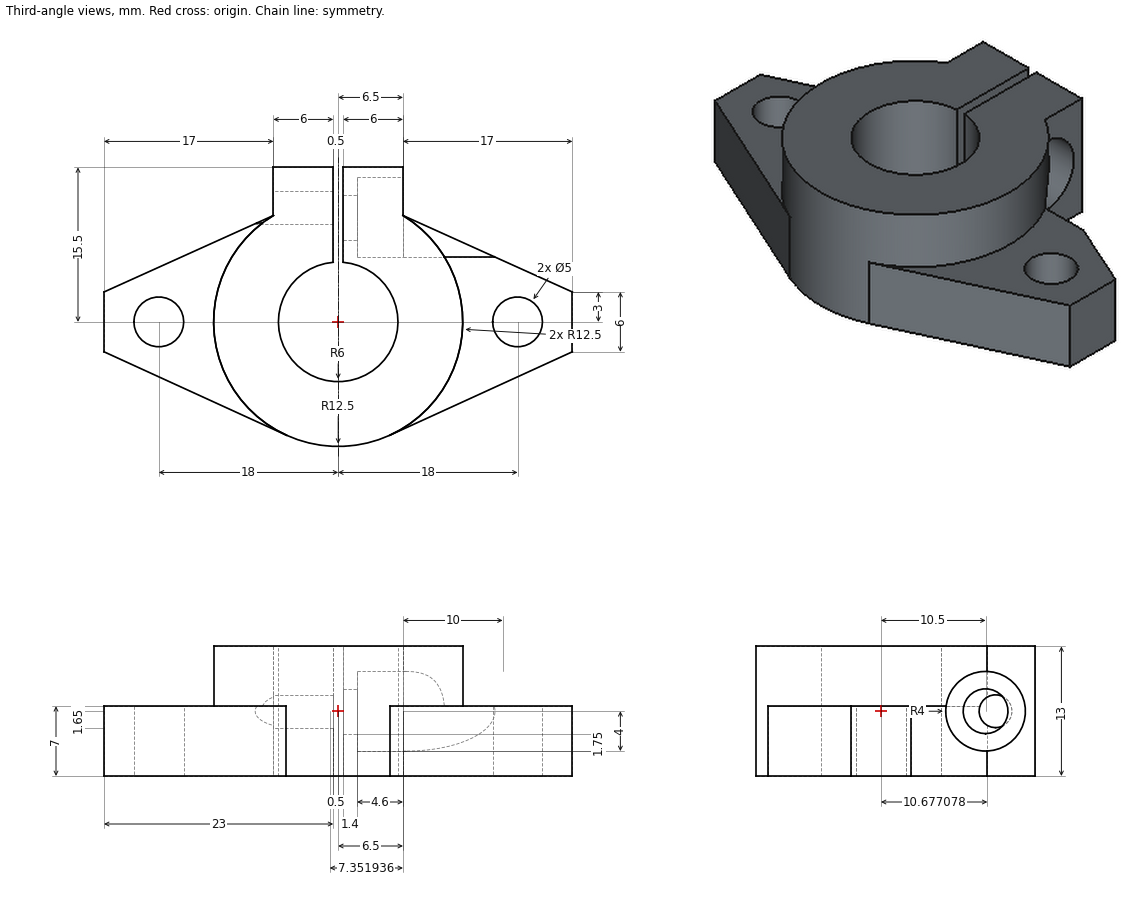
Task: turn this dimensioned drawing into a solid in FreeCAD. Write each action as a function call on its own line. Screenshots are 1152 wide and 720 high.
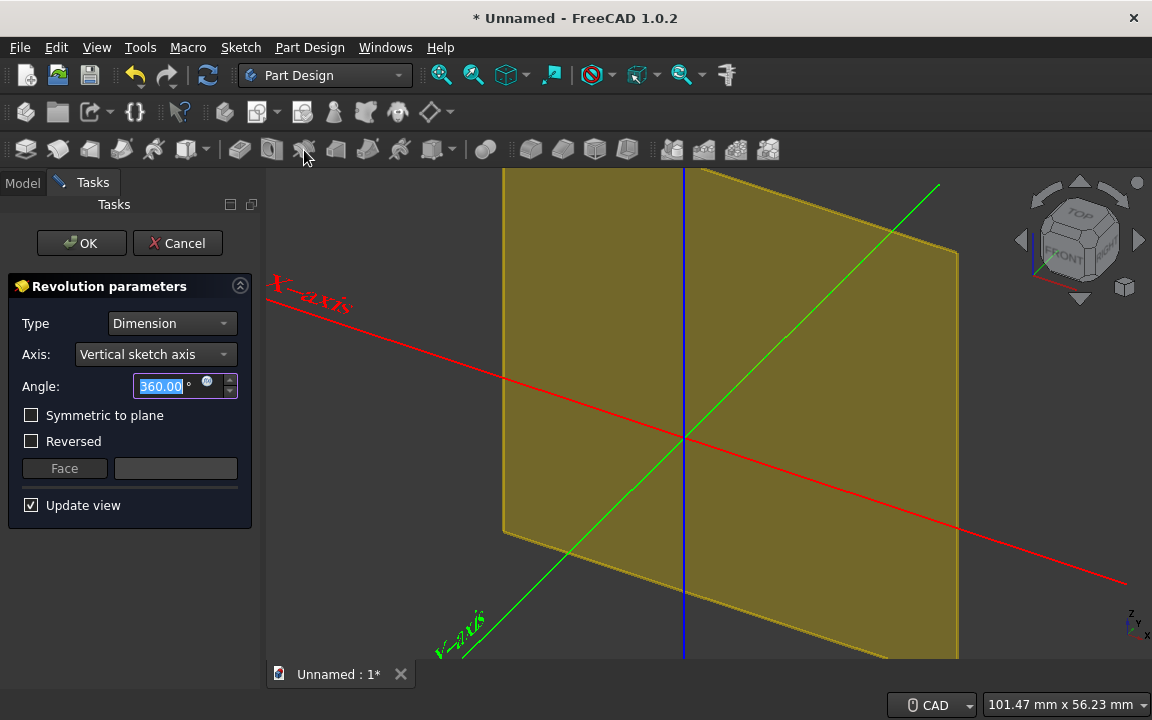
click(156, 354)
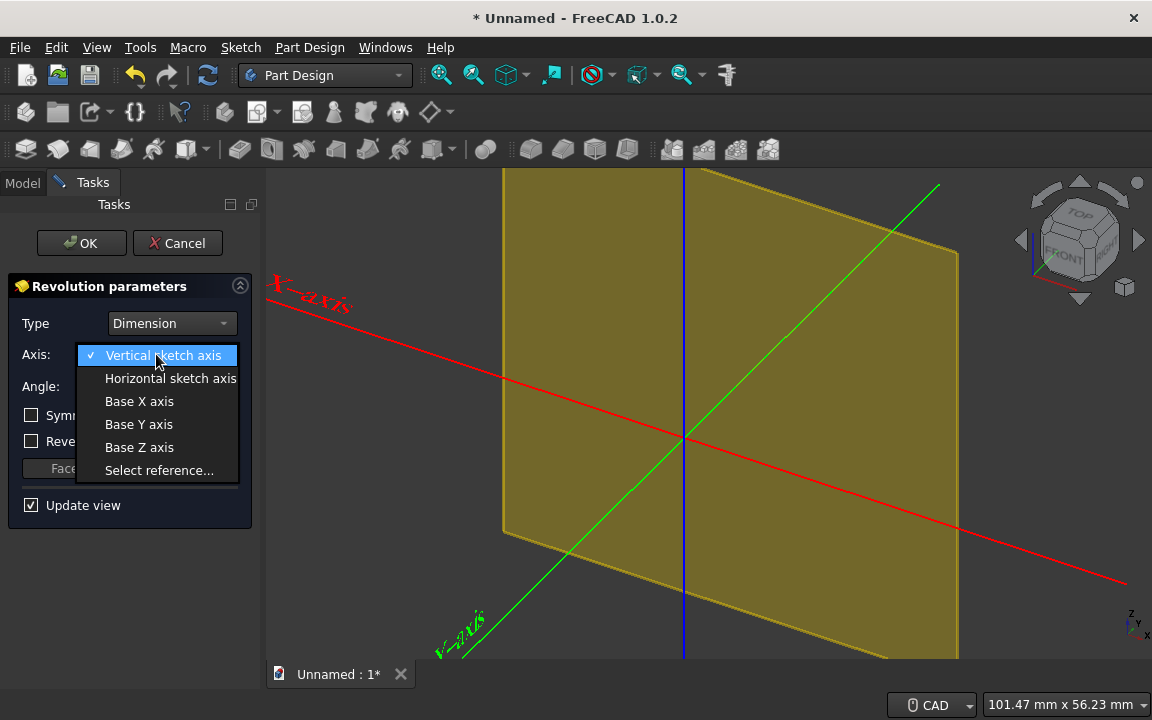
click(156, 378)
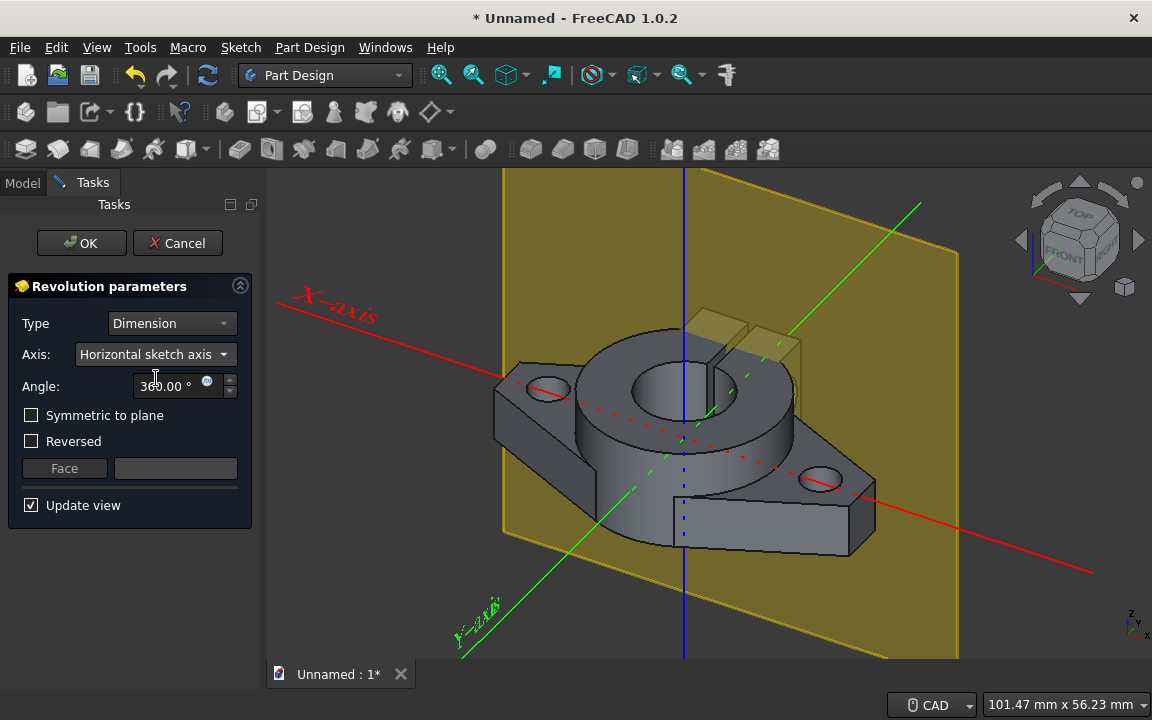
click(82, 243)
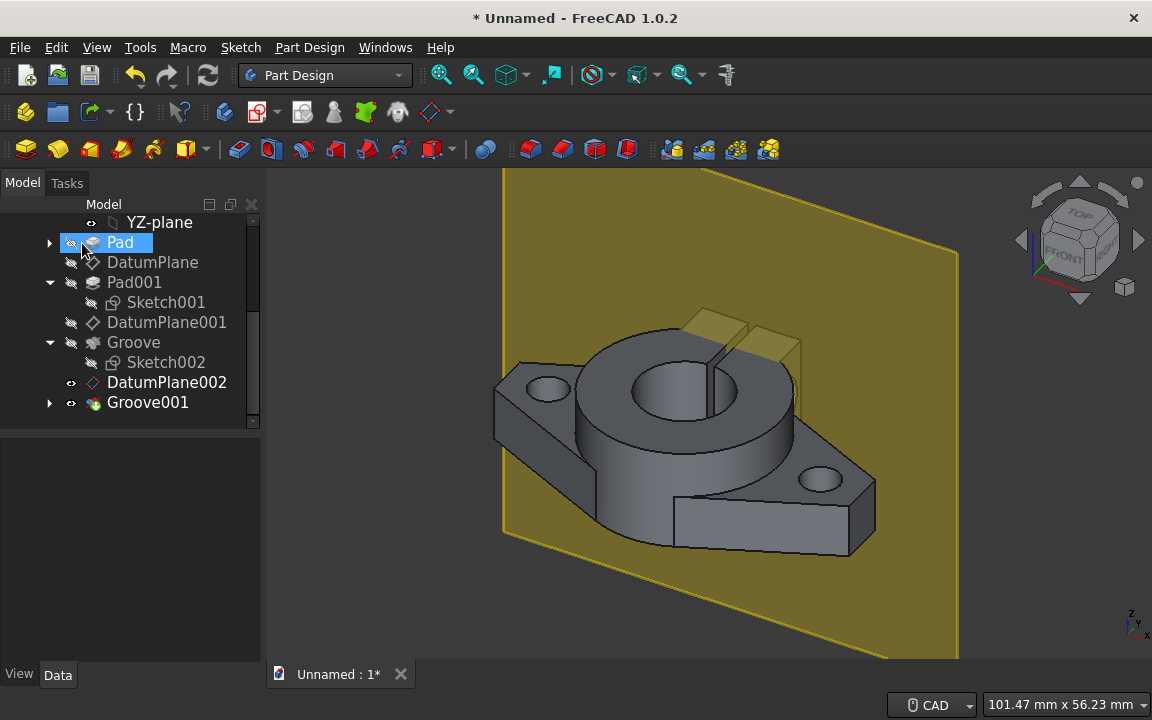
click(116, 383)
key(space)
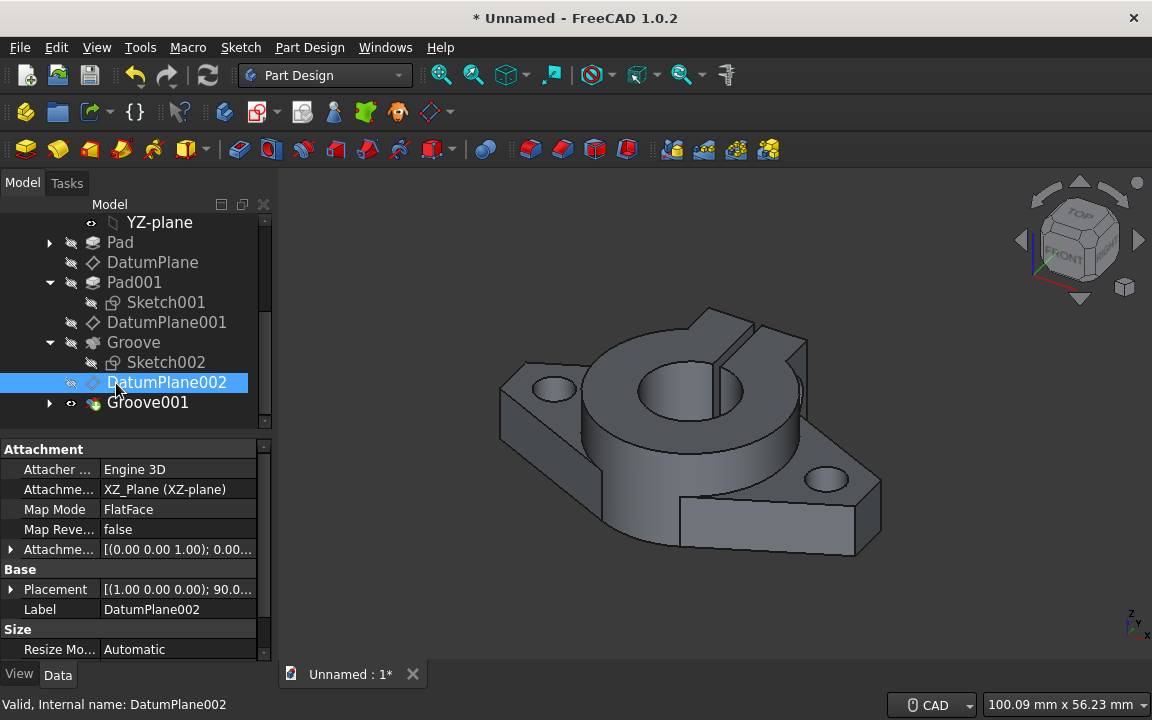
scroll(160, 318, down, 3)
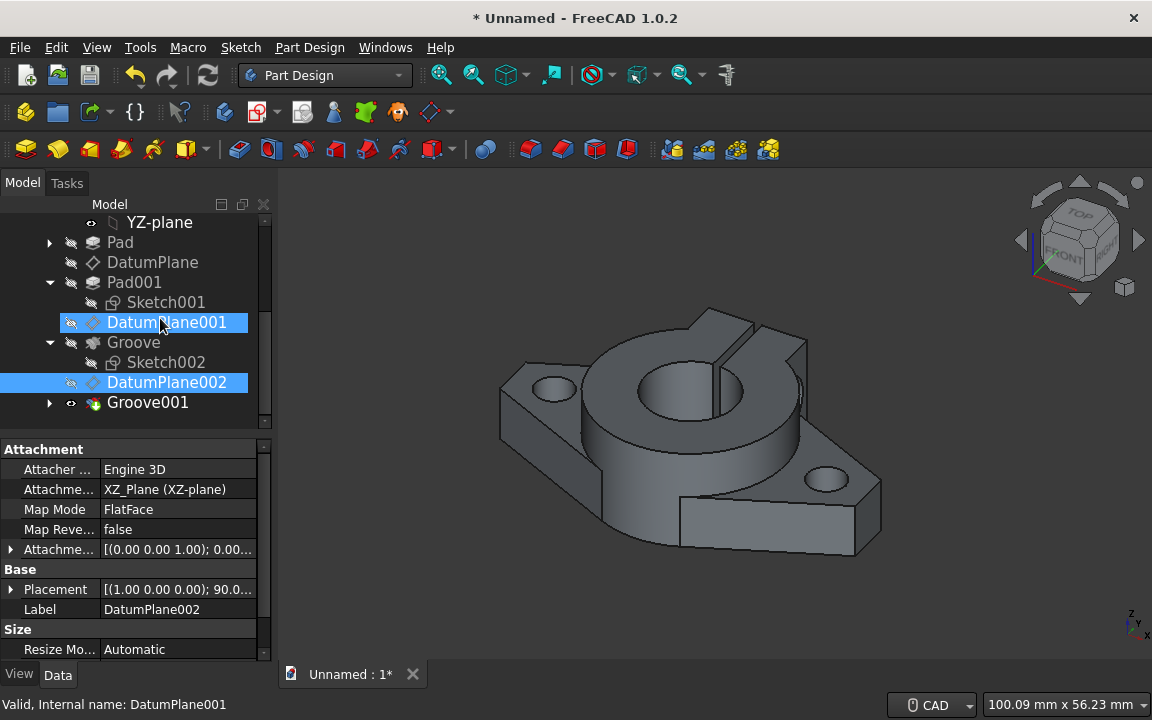
scroll(160, 318, up, 15)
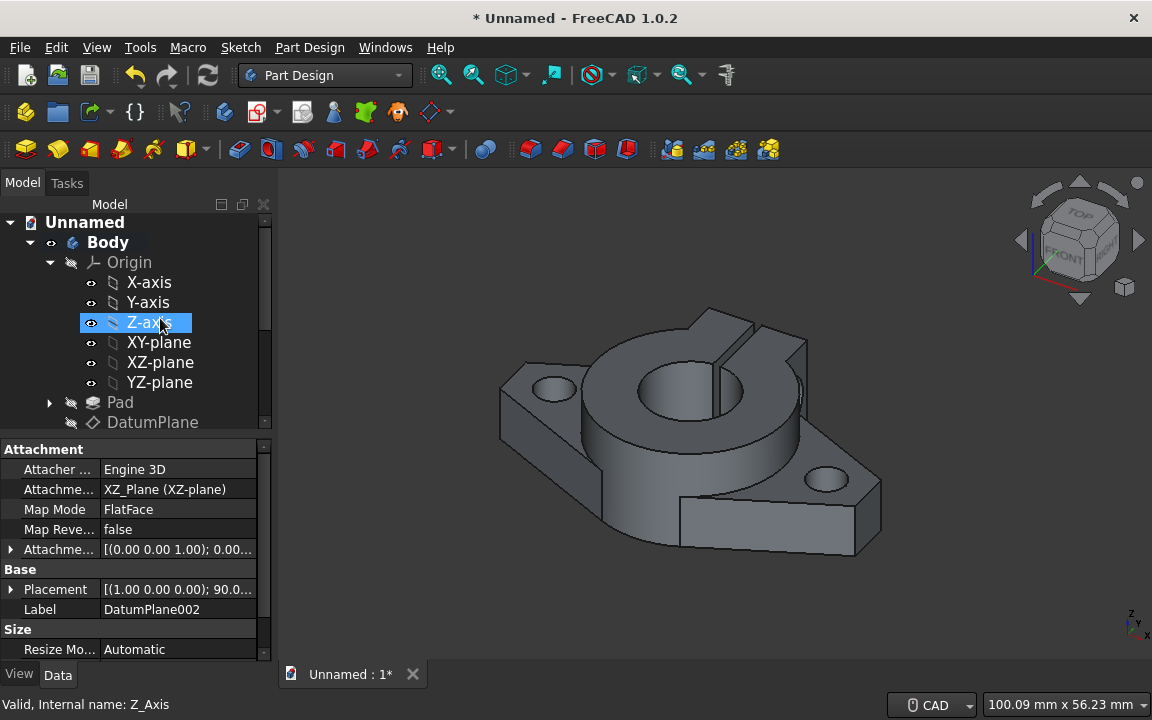
click(136, 383)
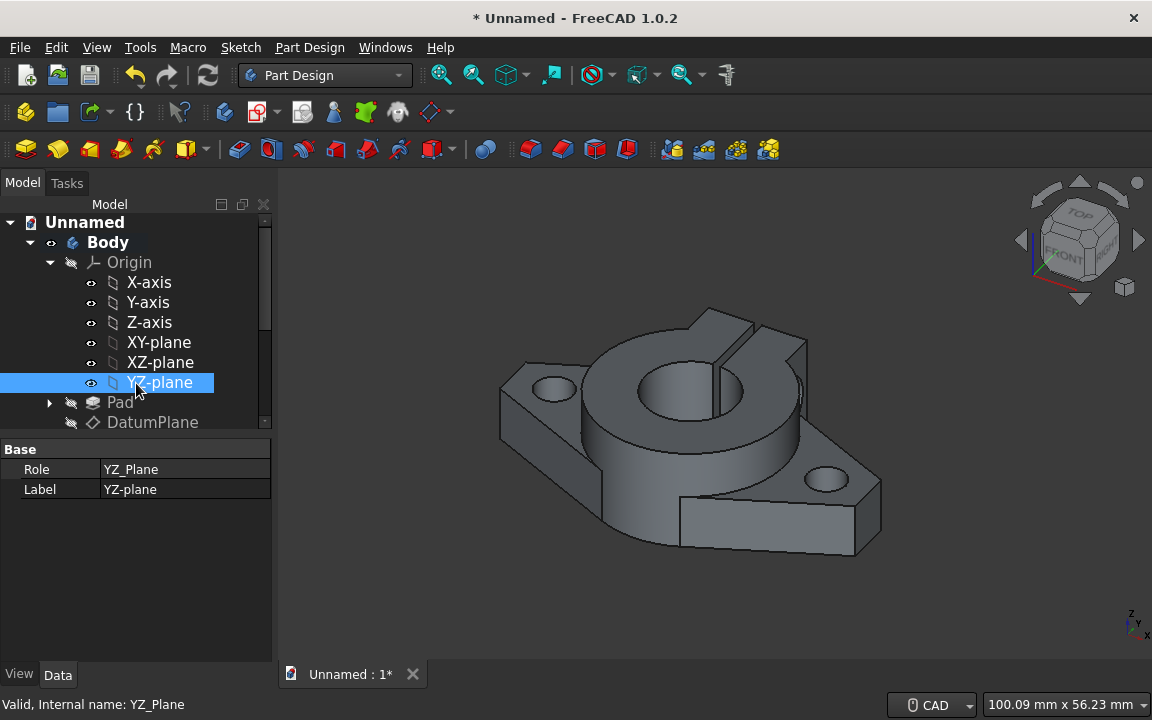
click(430, 112)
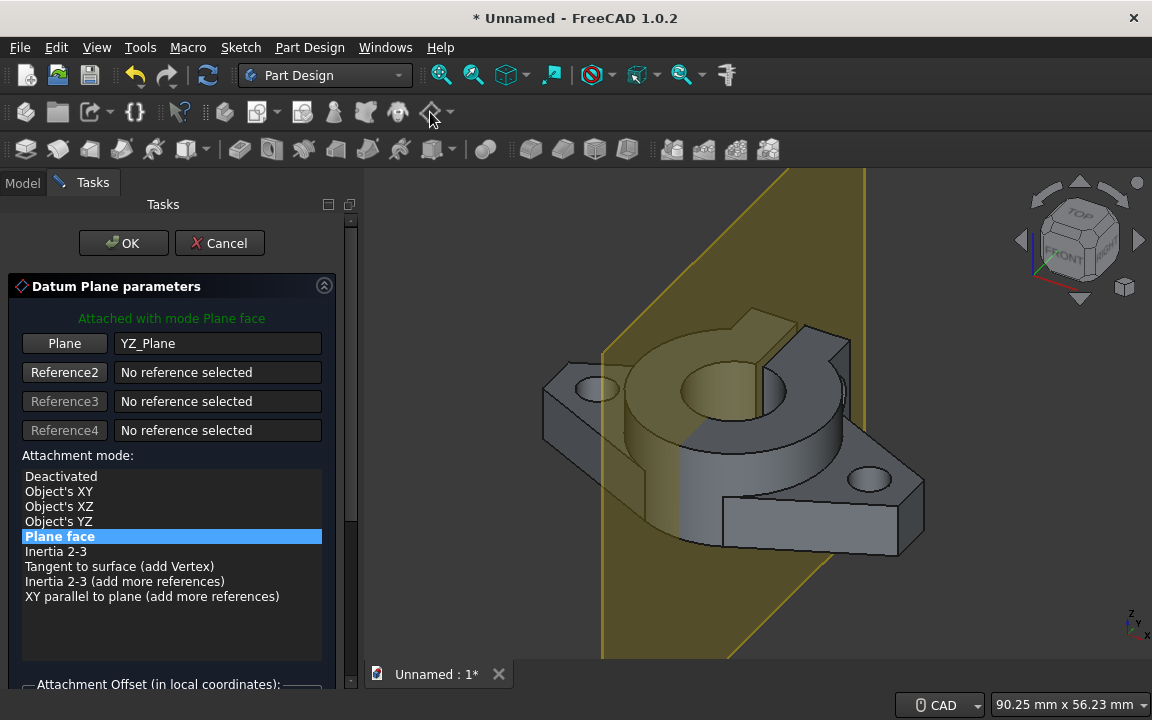
scroll(351, 451, down, 3)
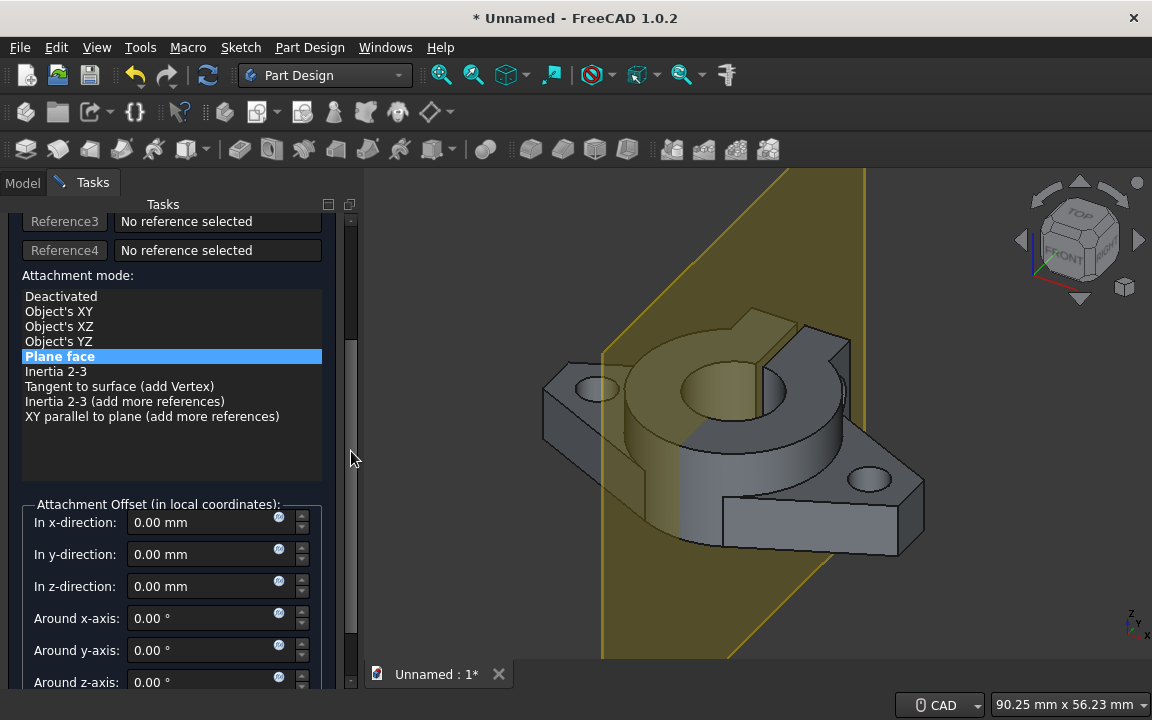
triple_click(210, 586)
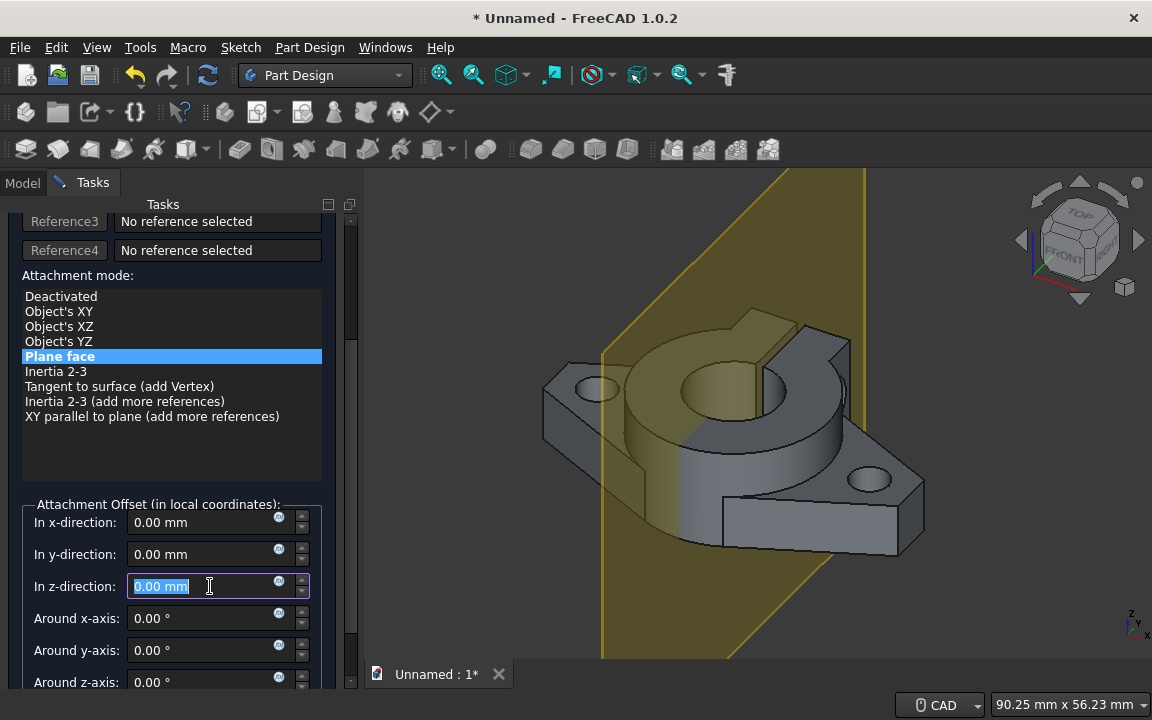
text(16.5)
key(Tab)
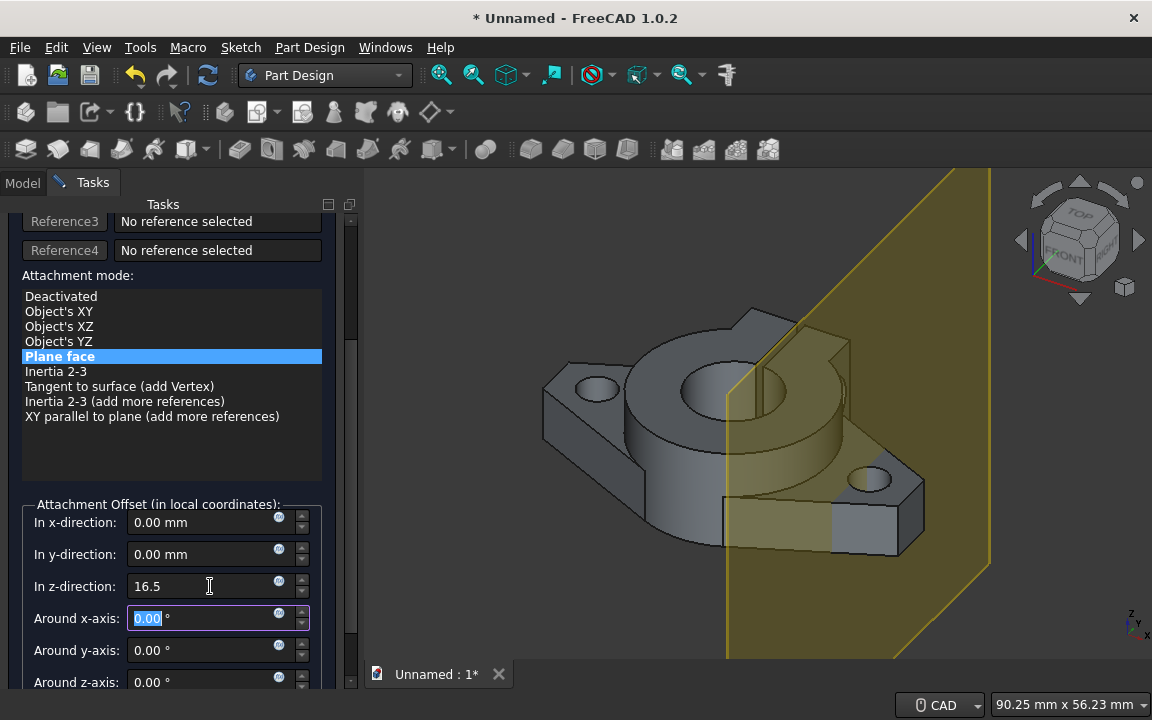
scroll(351, 451, up, 4)